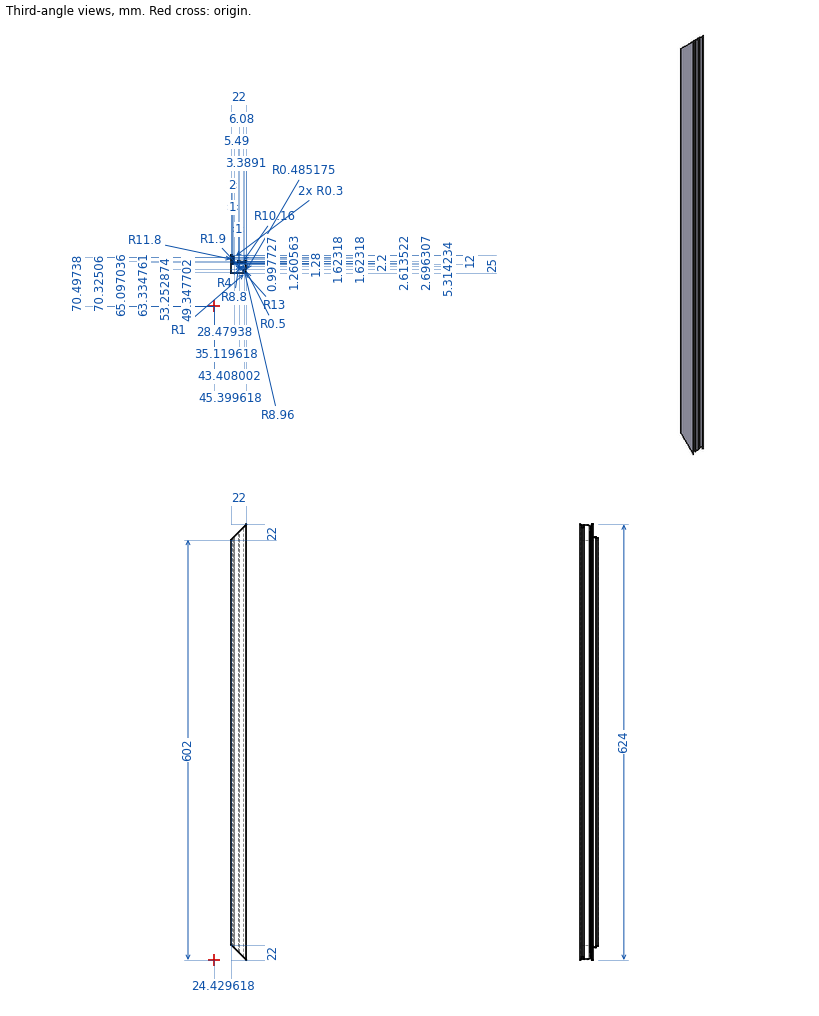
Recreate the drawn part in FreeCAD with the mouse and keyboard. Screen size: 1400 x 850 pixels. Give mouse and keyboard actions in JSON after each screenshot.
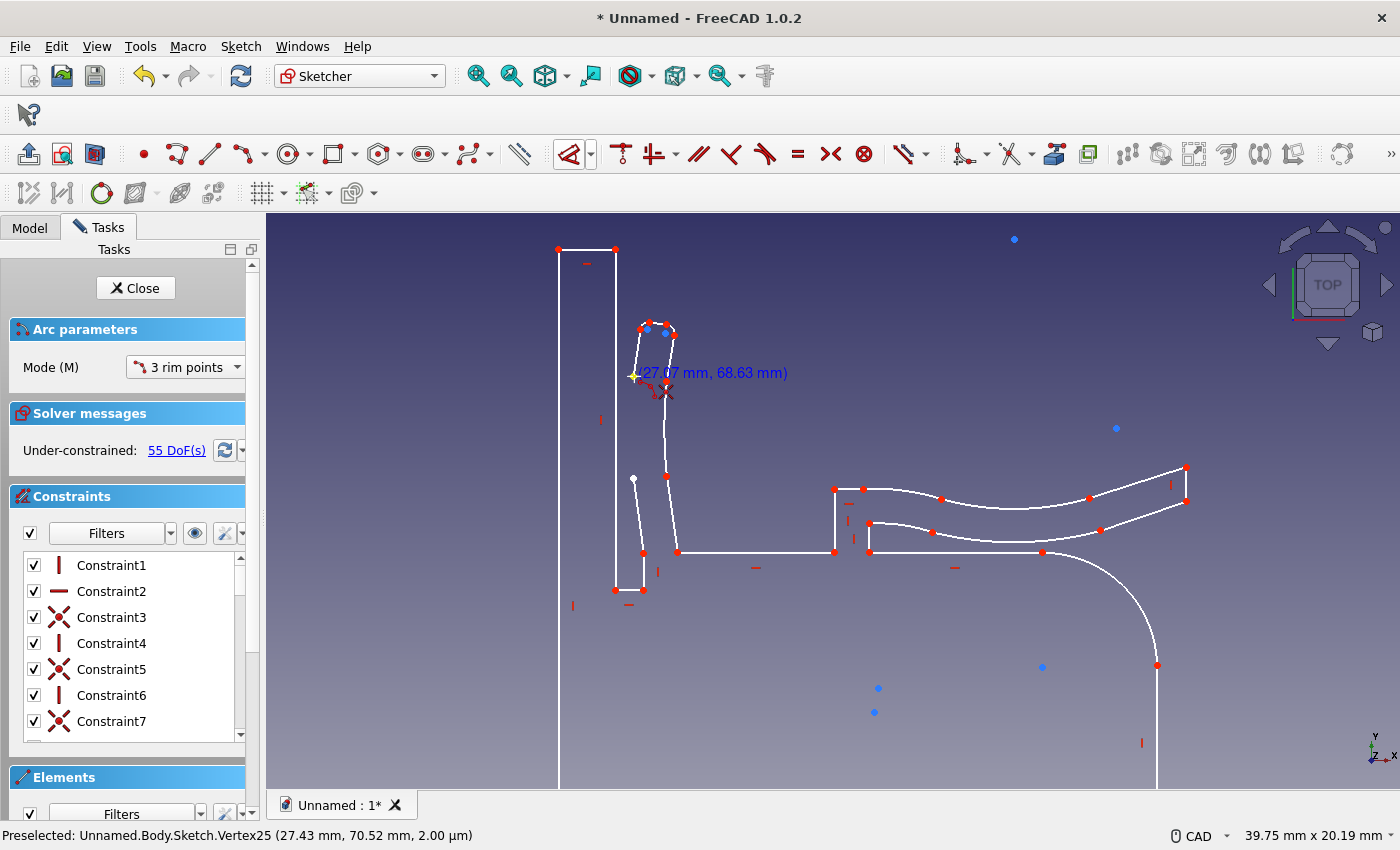
{"action": "left_click", "coordinate": [634, 376]}
{"action": "left_click", "coordinate": [634, 479]}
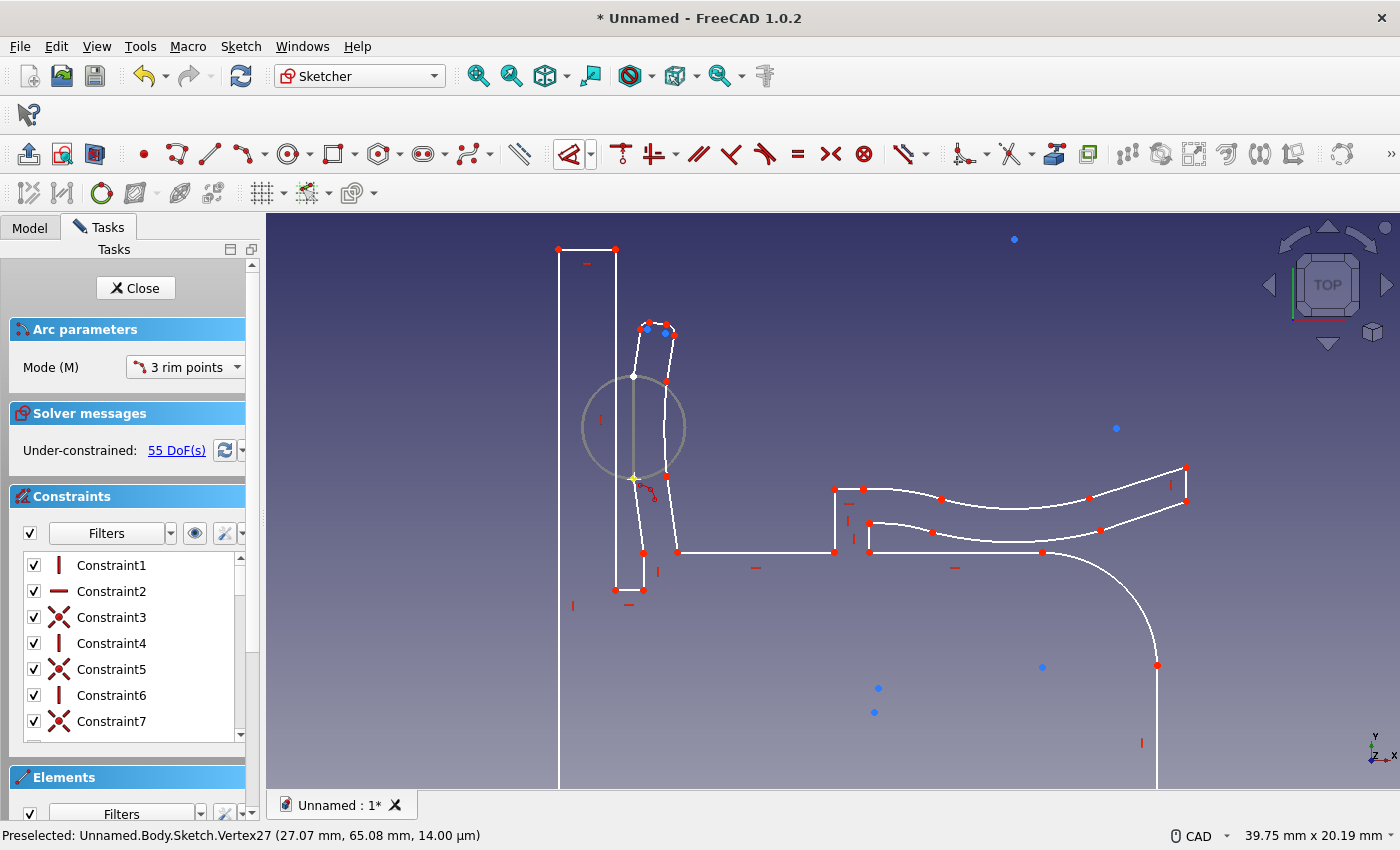
{"action": "scroll", "coordinate": [630, 427], "scroll_direction": "up", "scroll_amount": 8}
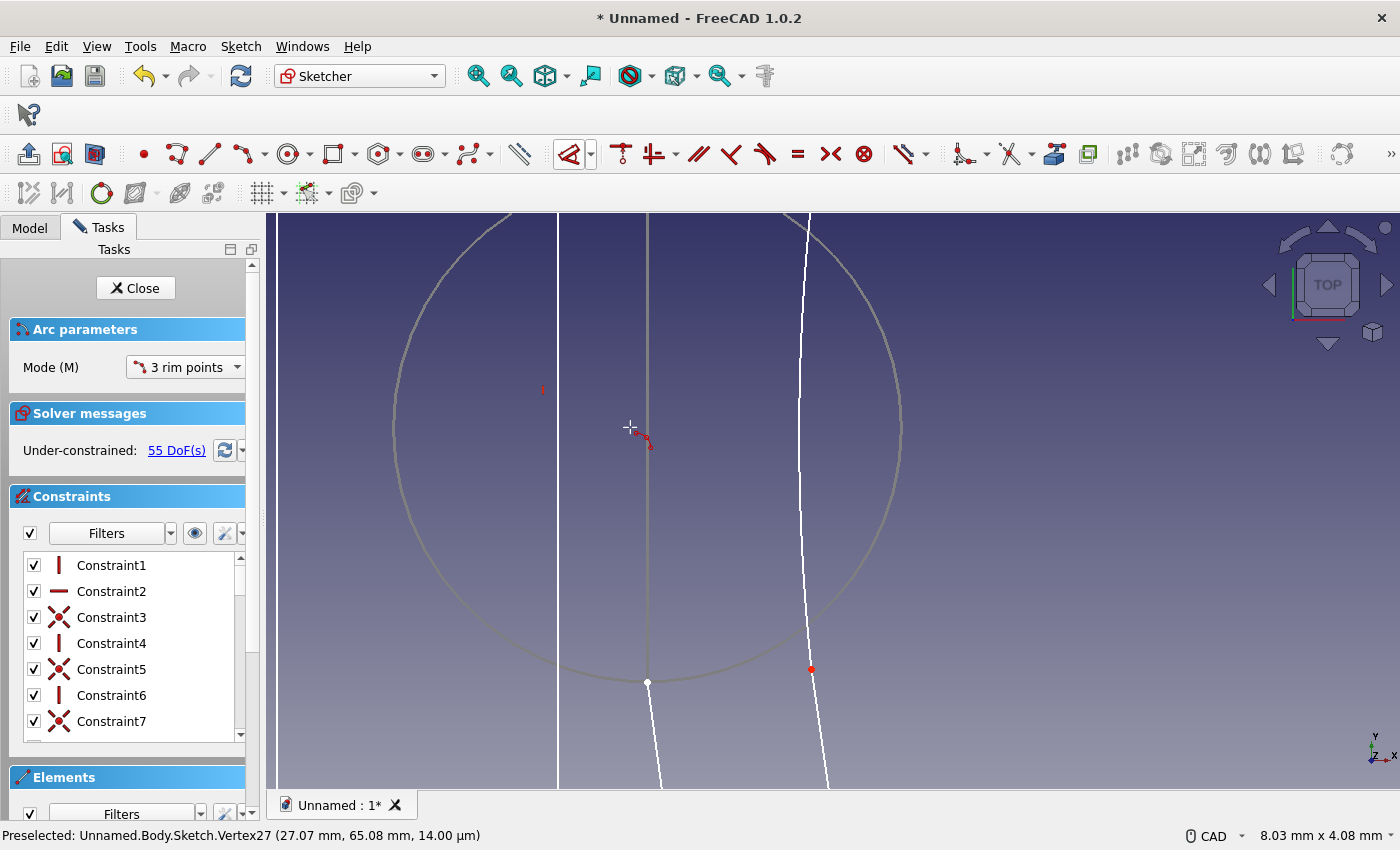
{"action": "left_click", "coordinate": [629, 425]}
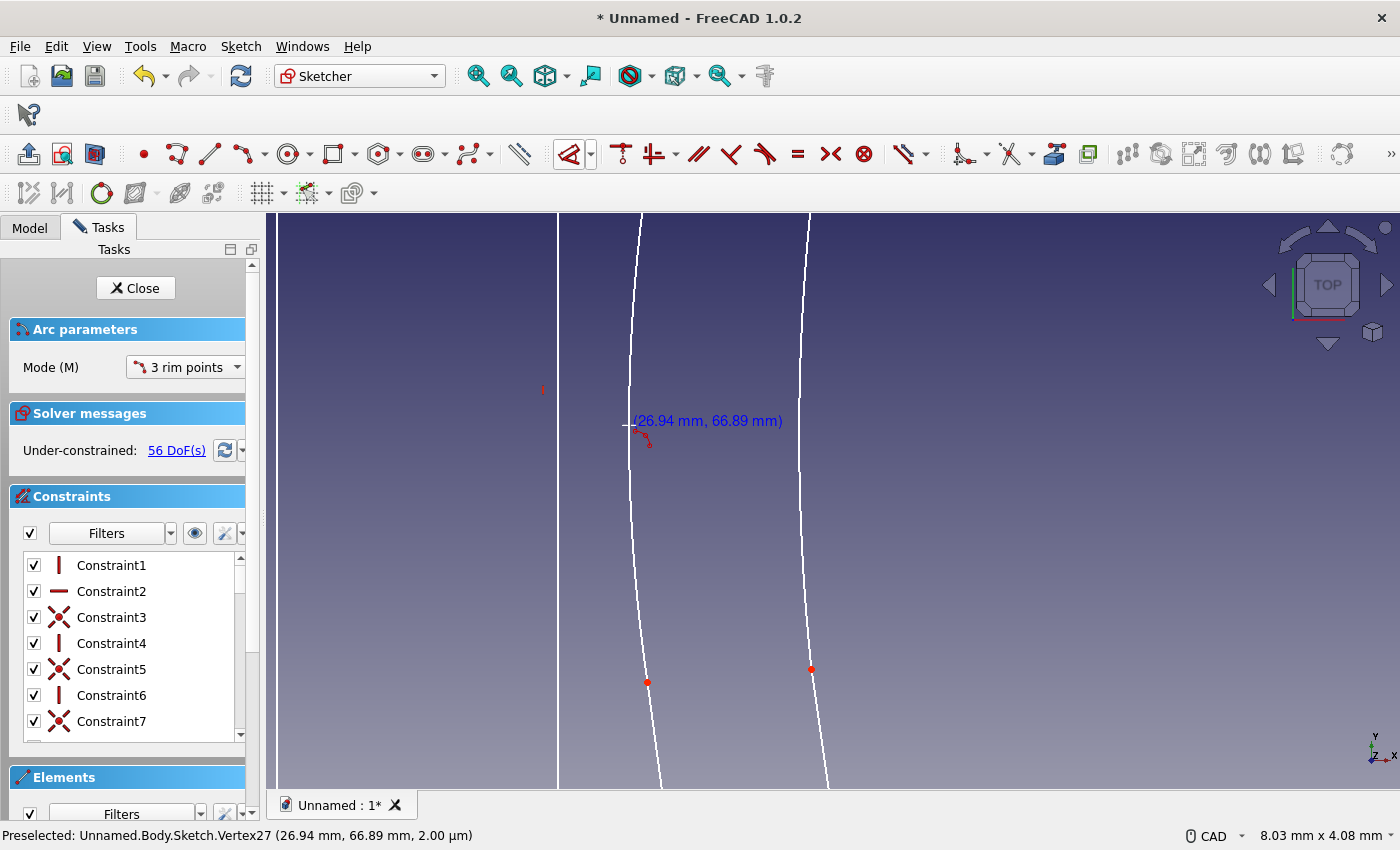
{"action": "scroll", "coordinate": [632, 401], "scroll_direction": "down", "scroll_amount": 11}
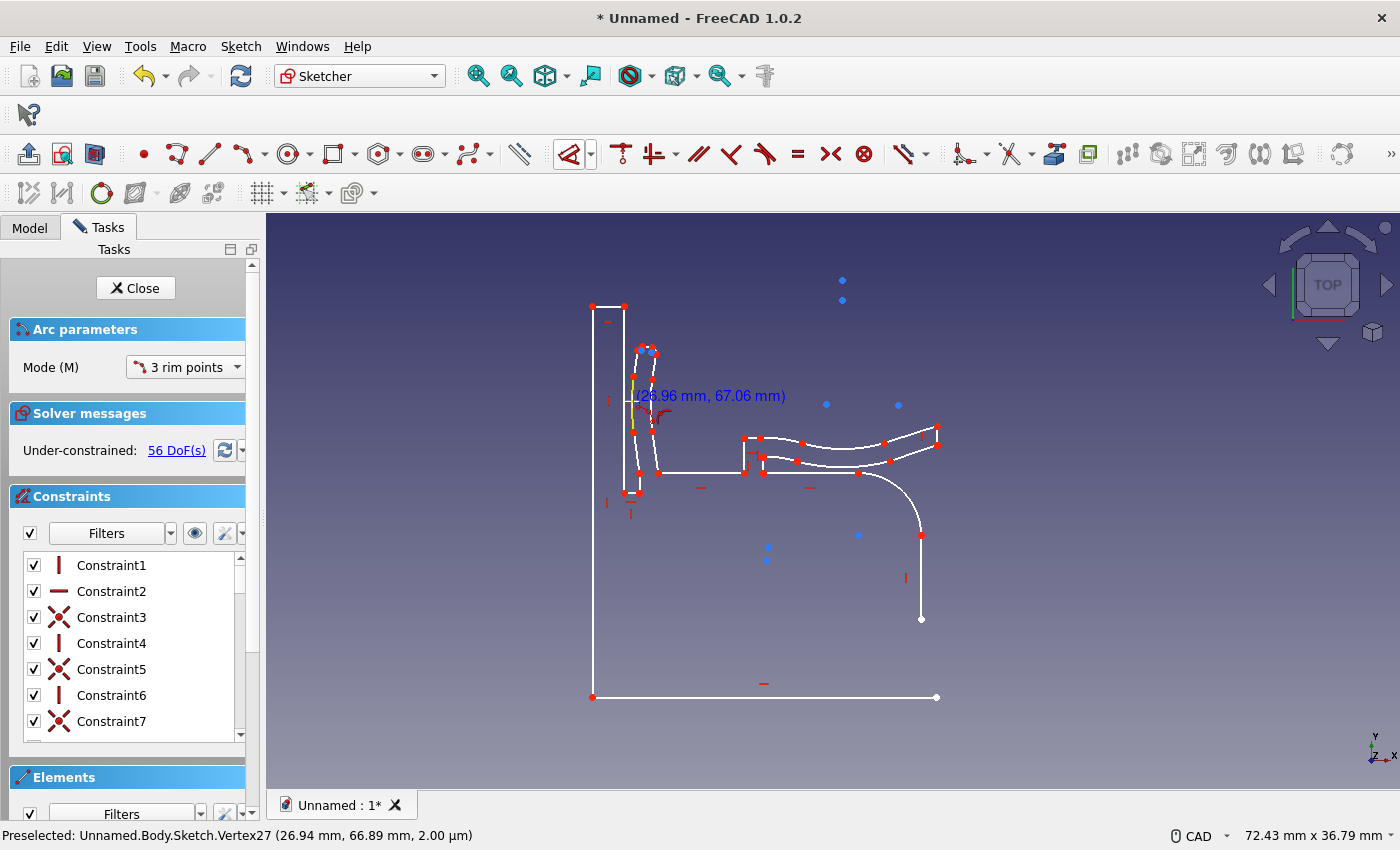
{"action": "left_click", "coordinate": [937, 698]}
{"action": "left_click", "coordinate": [922, 679]}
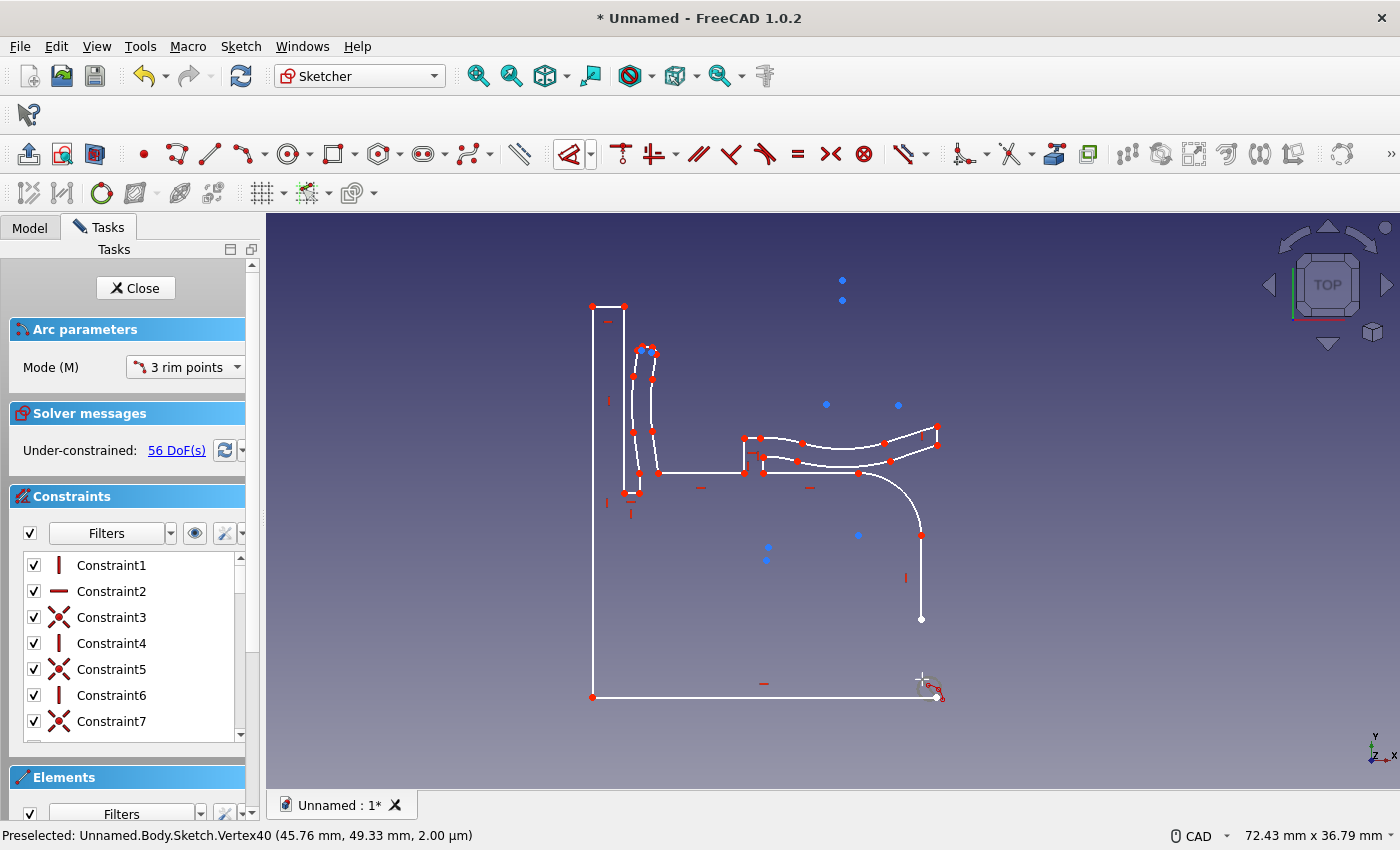
{"action": "scroll", "coordinate": [925, 691], "scroll_direction": "up", "scroll_amount": 6}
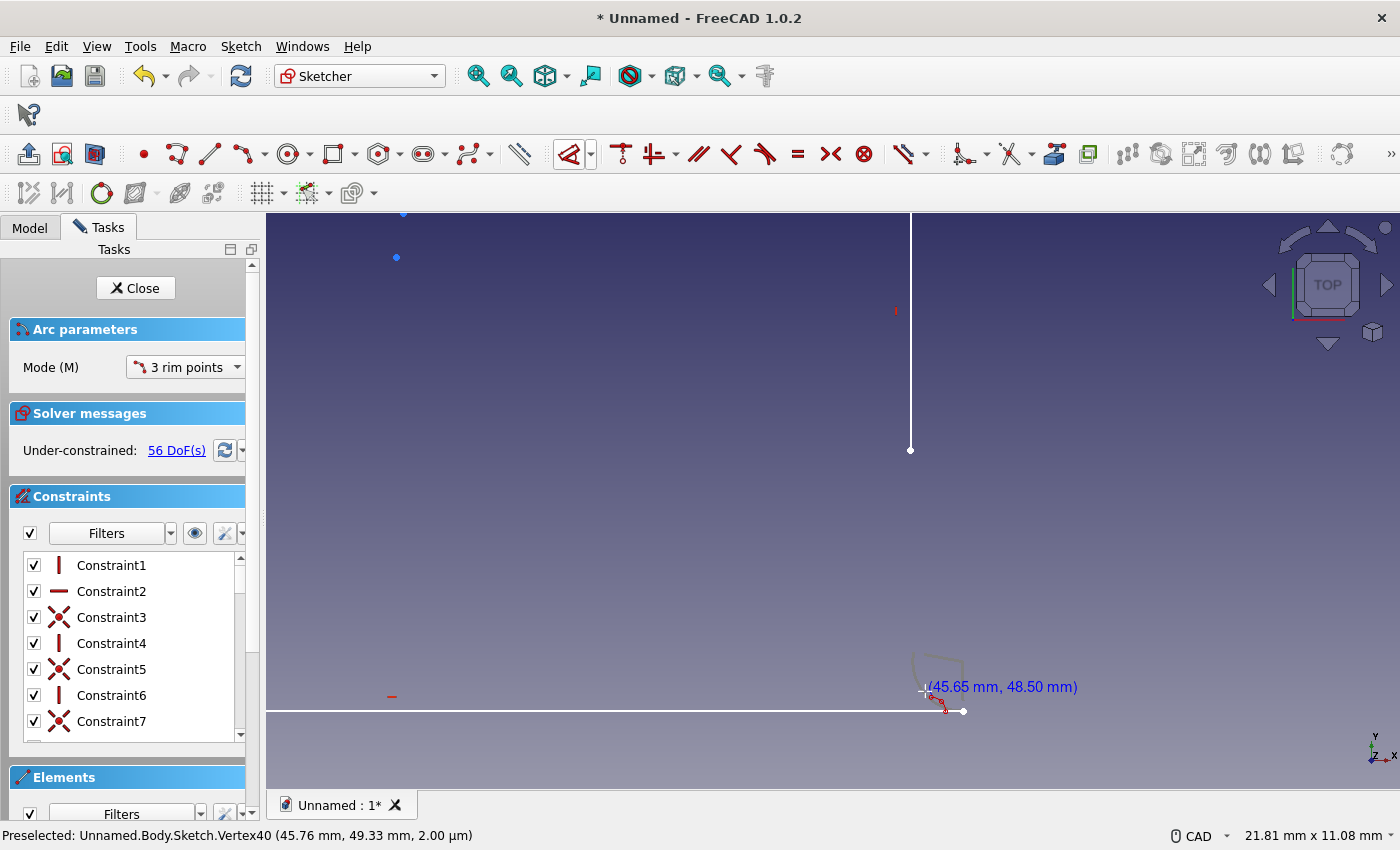
{"action": "left_click", "coordinate": [925, 690]}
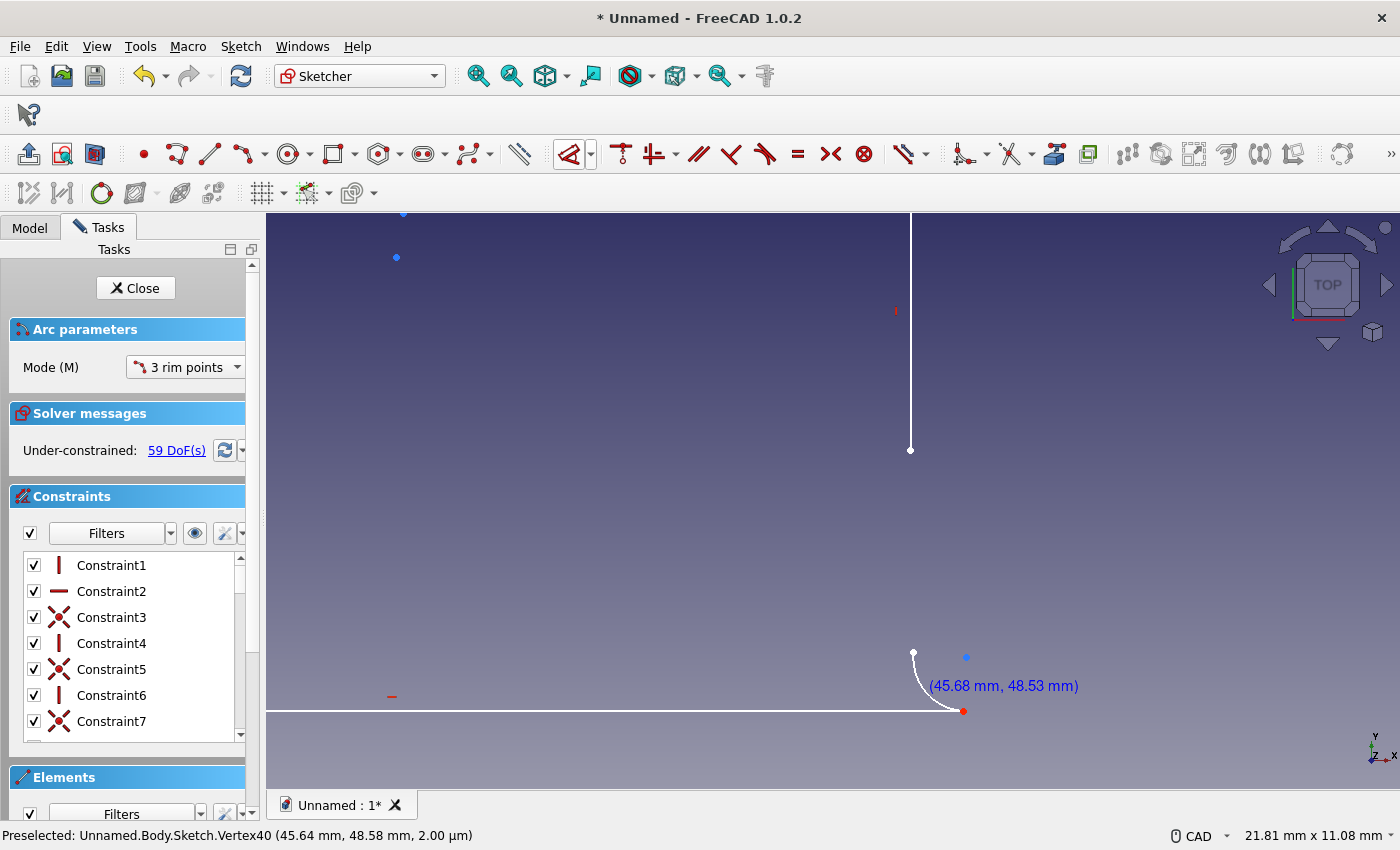
{"action": "left_click", "coordinate": [914, 653]}
{"action": "left_click", "coordinate": [872, 625]}
{"action": "left_click", "coordinate": [900, 623]}